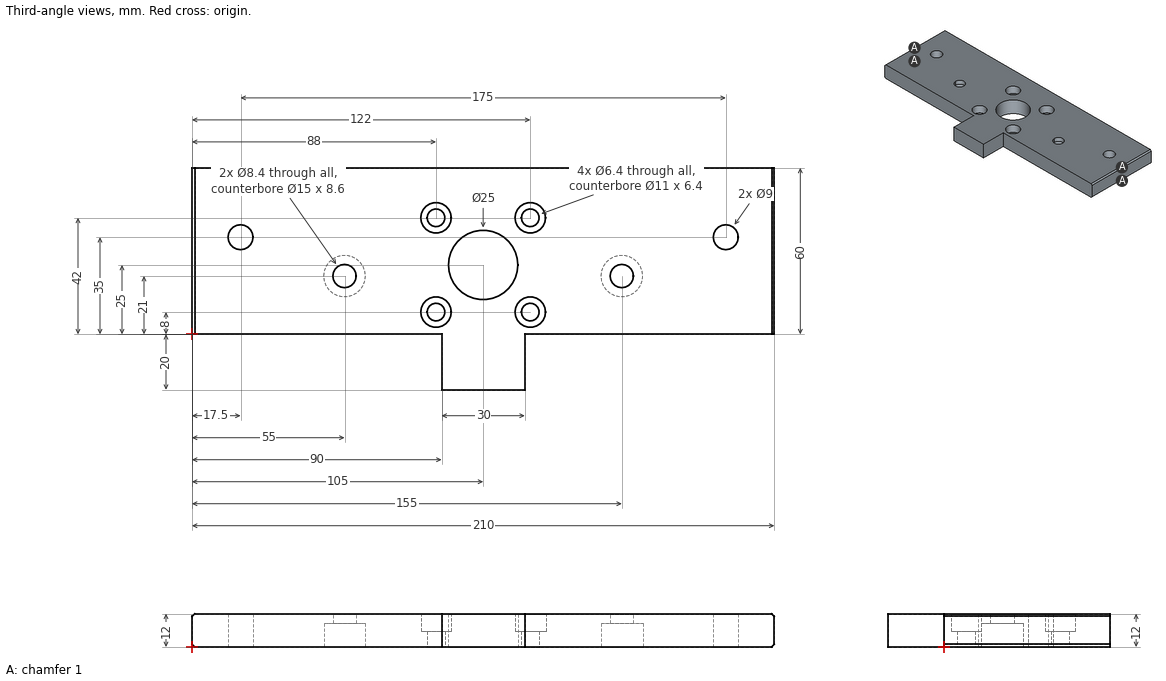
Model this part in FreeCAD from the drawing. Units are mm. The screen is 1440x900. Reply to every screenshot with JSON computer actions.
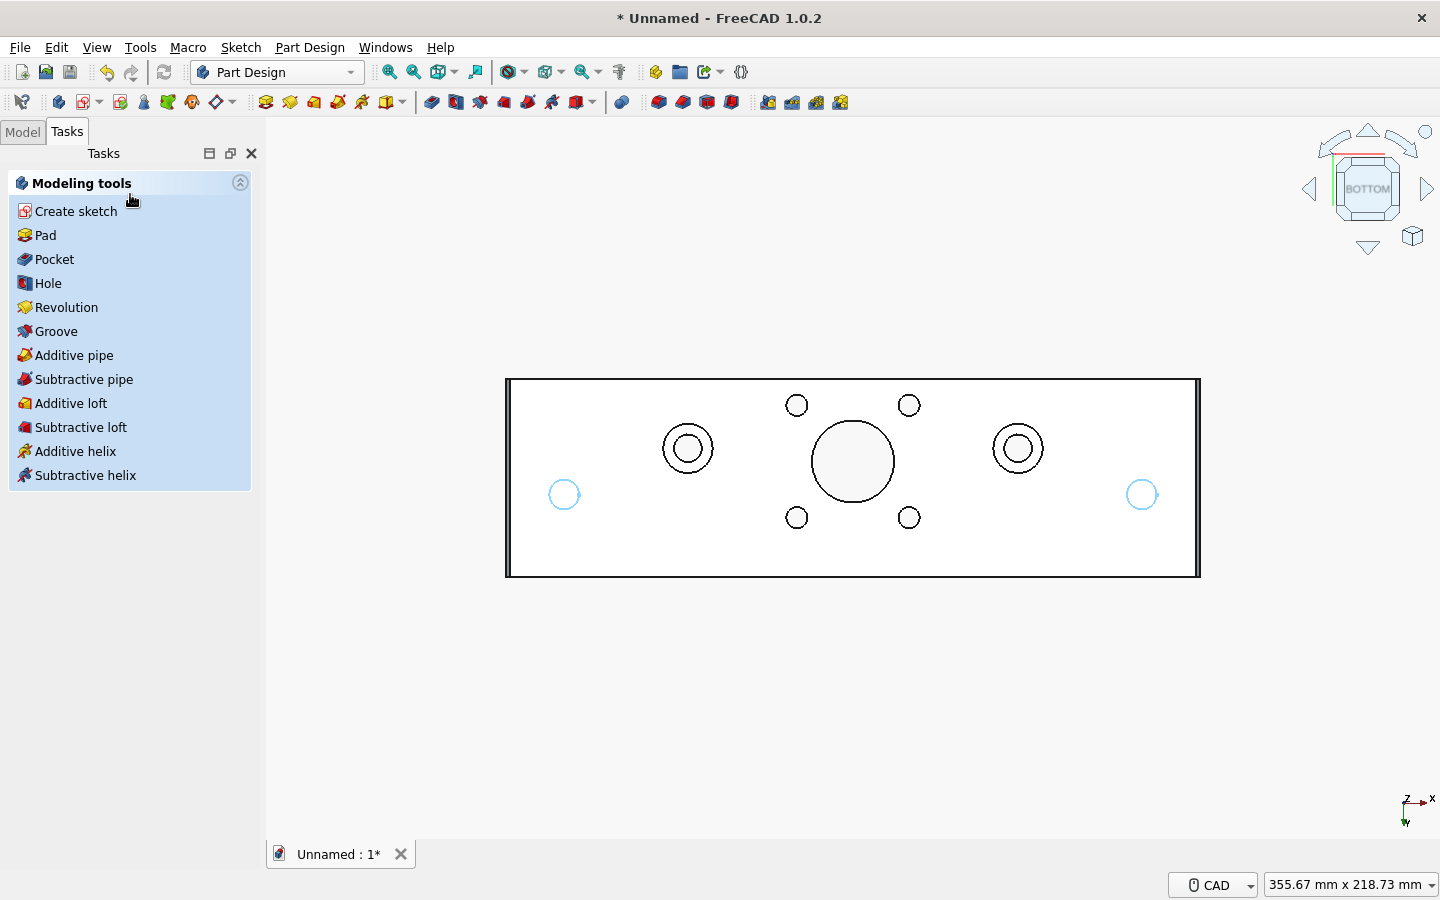
{"action": "left_click", "coordinate": [432, 102]}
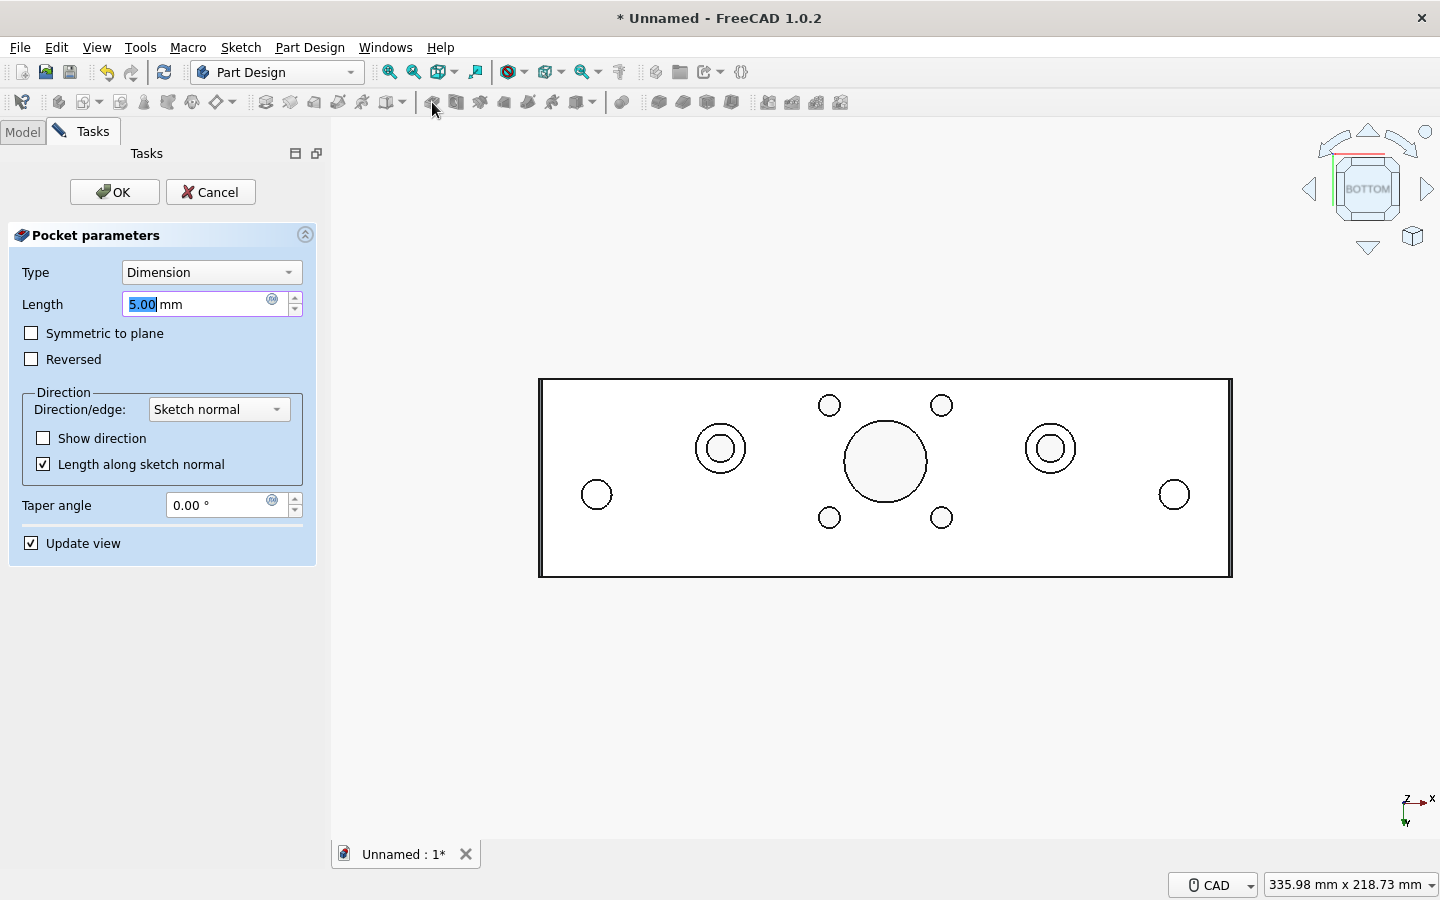
{"action": "left_click", "coordinate": [212, 272]}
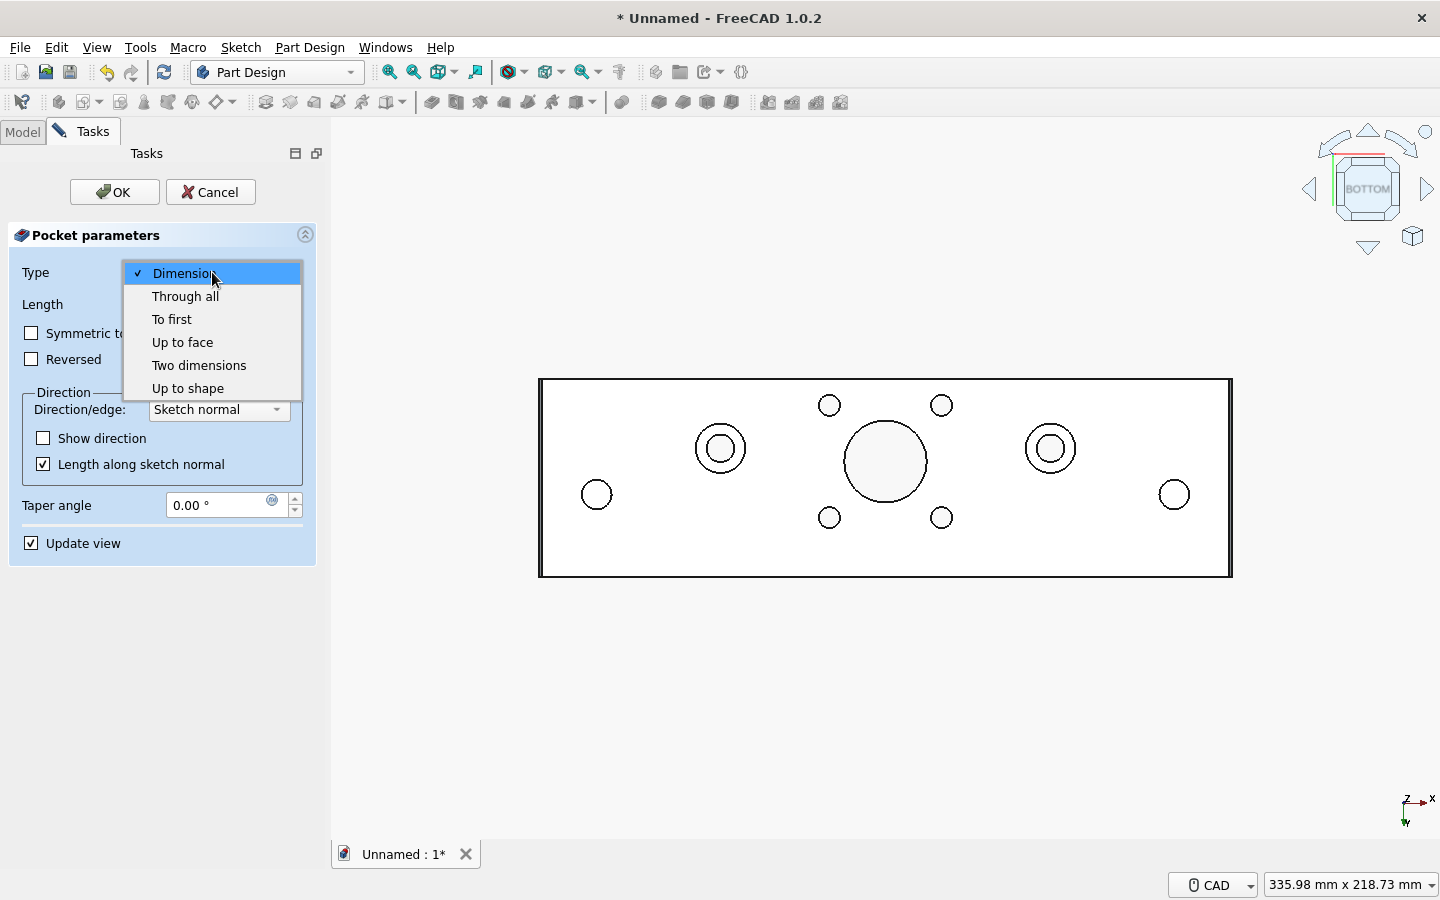
{"action": "left_click", "coordinate": [212, 296]}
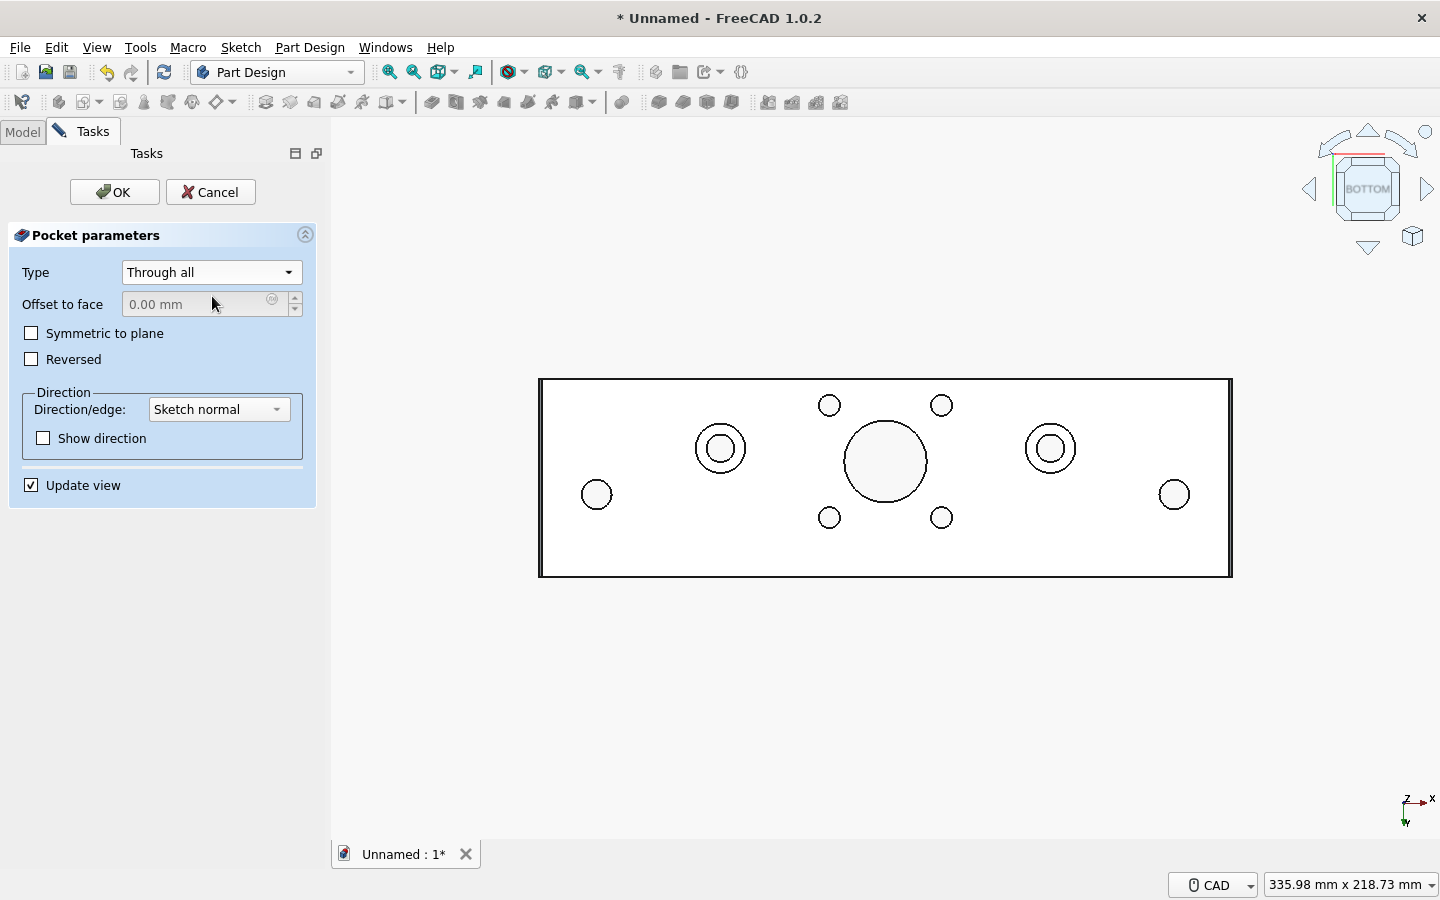
{"action": "left_click", "coordinate": [115, 192]}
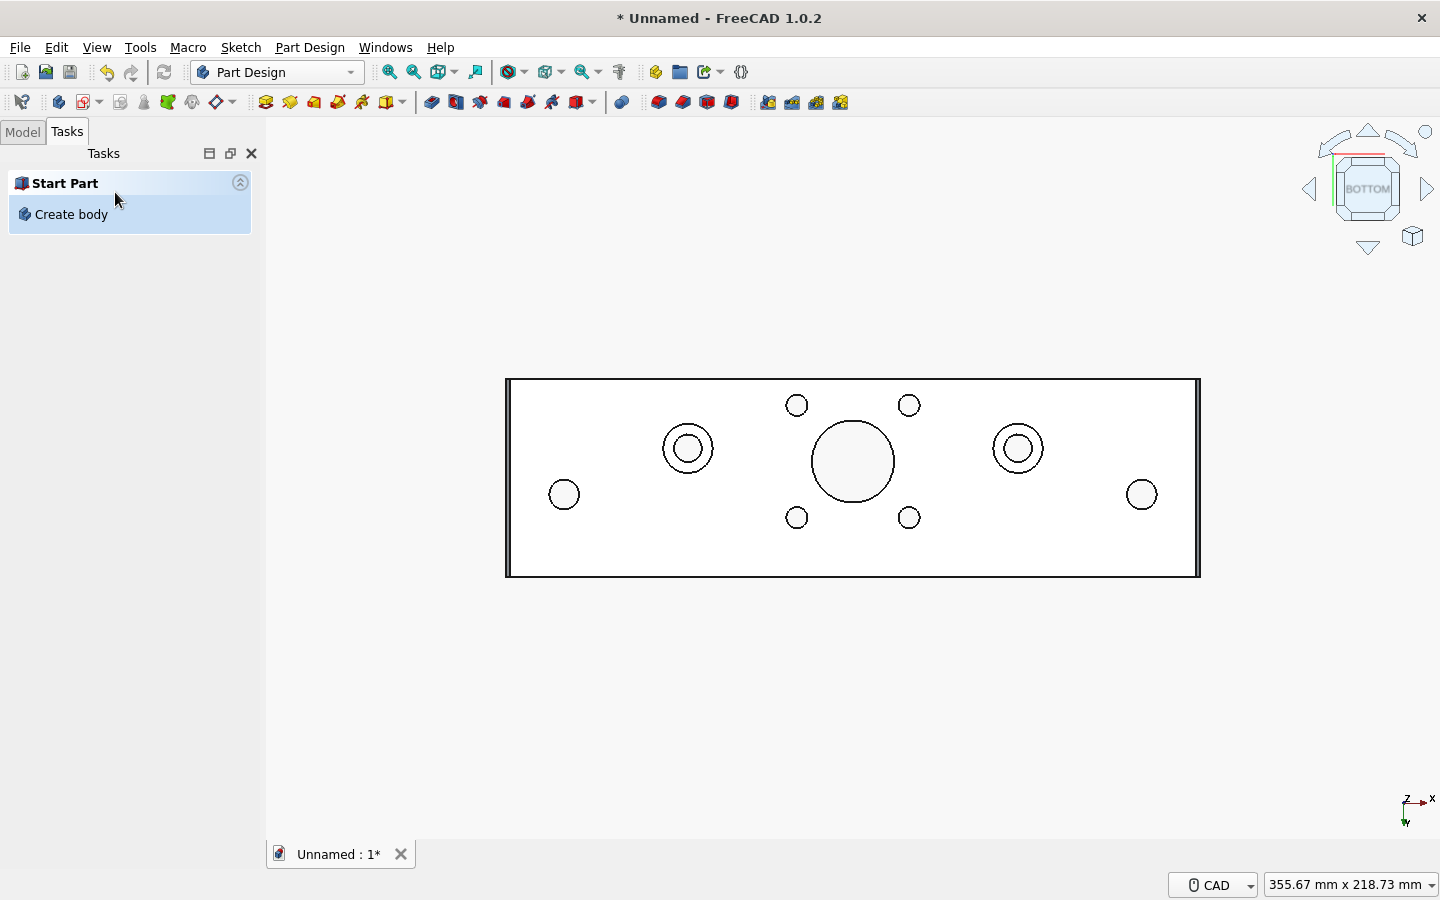
{"action": "left_click", "coordinate": [951, 477]}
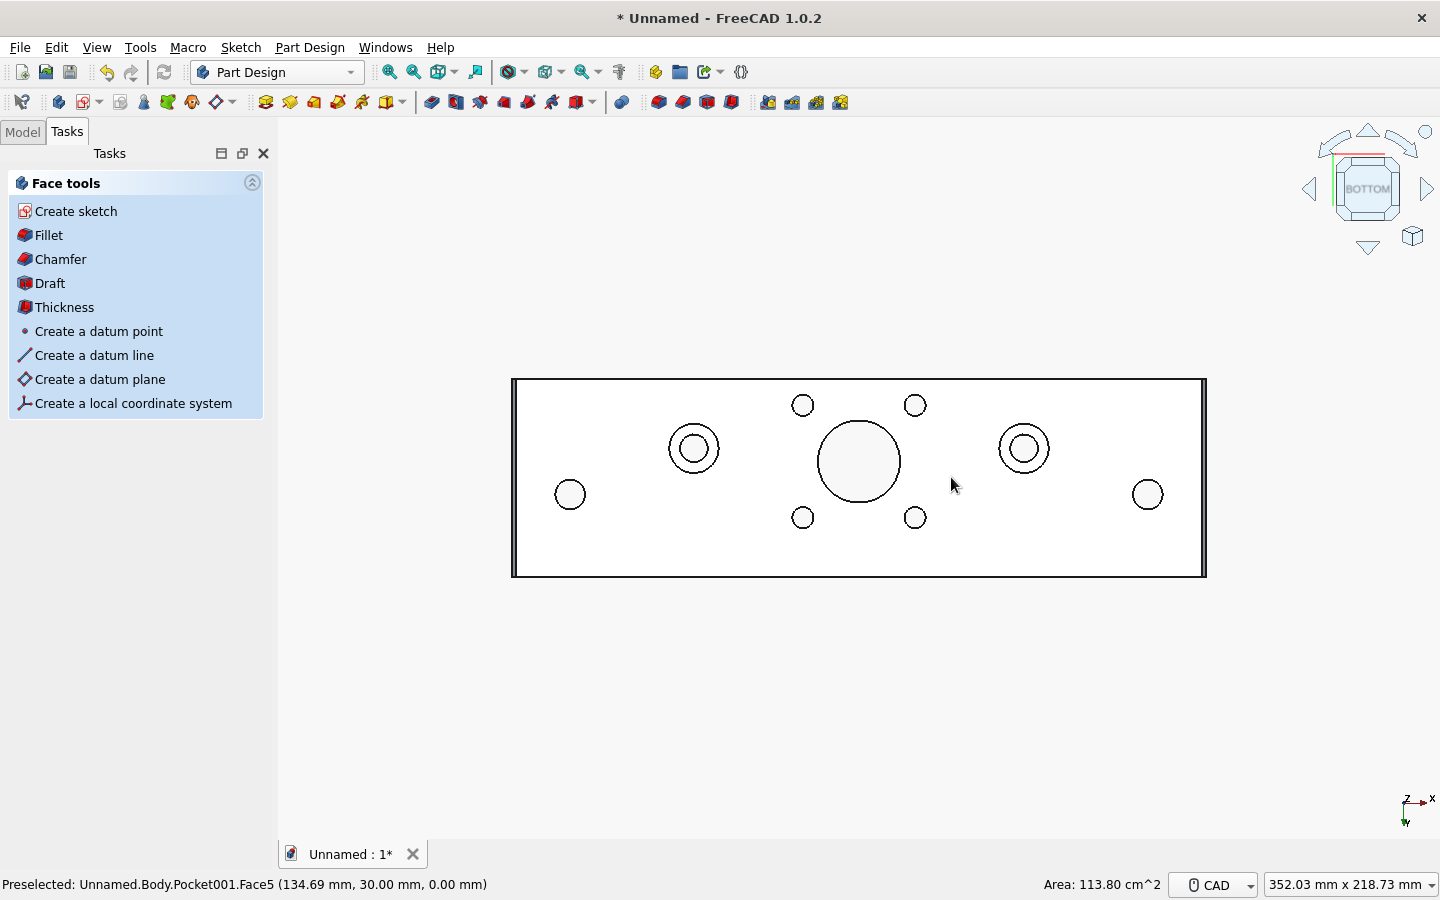
{"action": "left_click", "coordinate": [84, 102]}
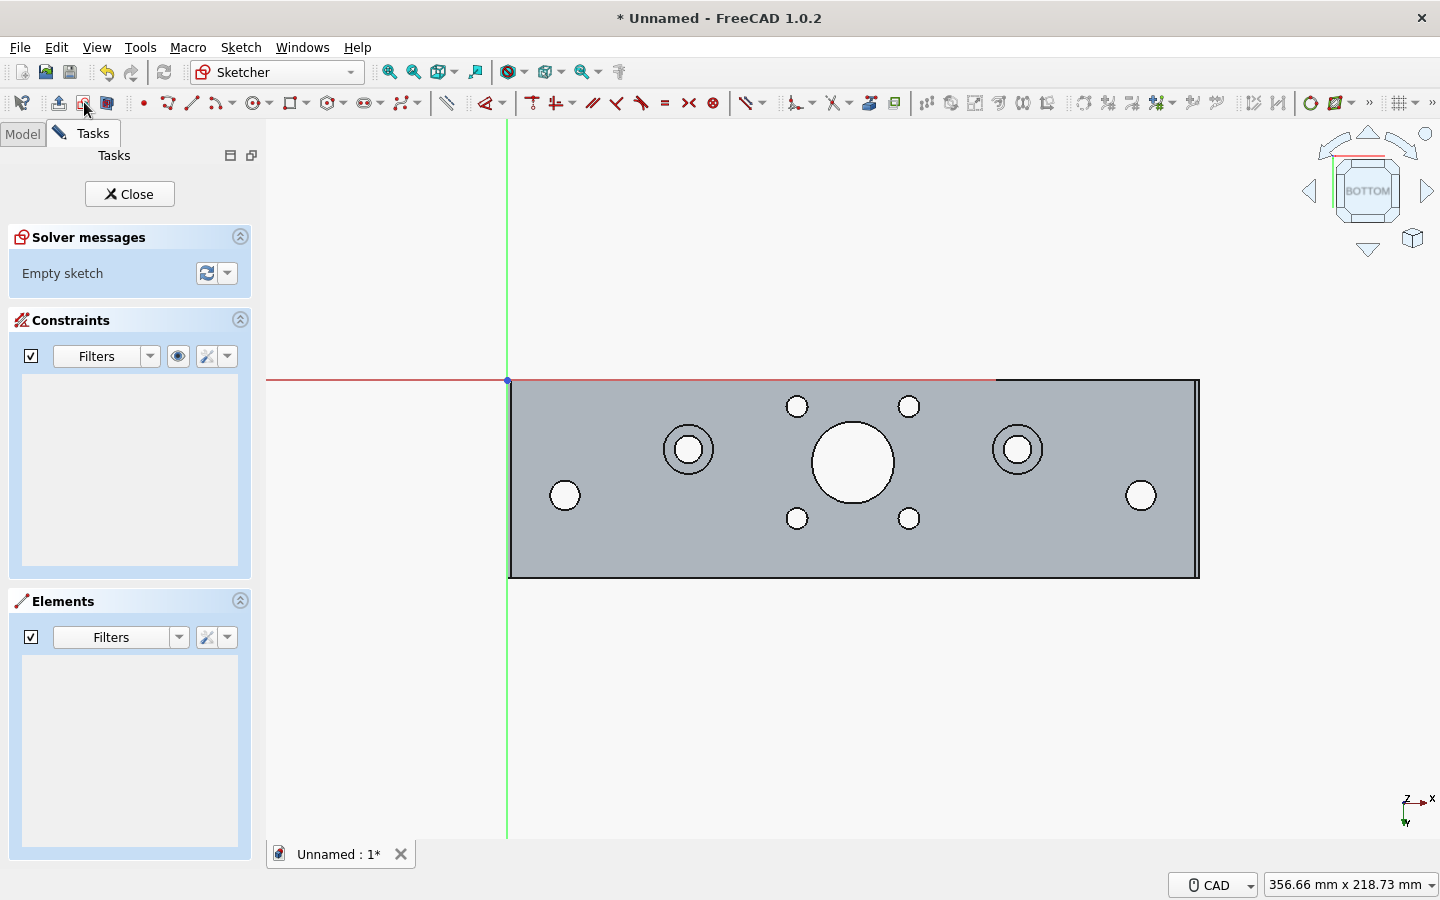
{"action": "scroll", "coordinate": [864, 327], "scroll_direction": "up", "scroll_amount": 10}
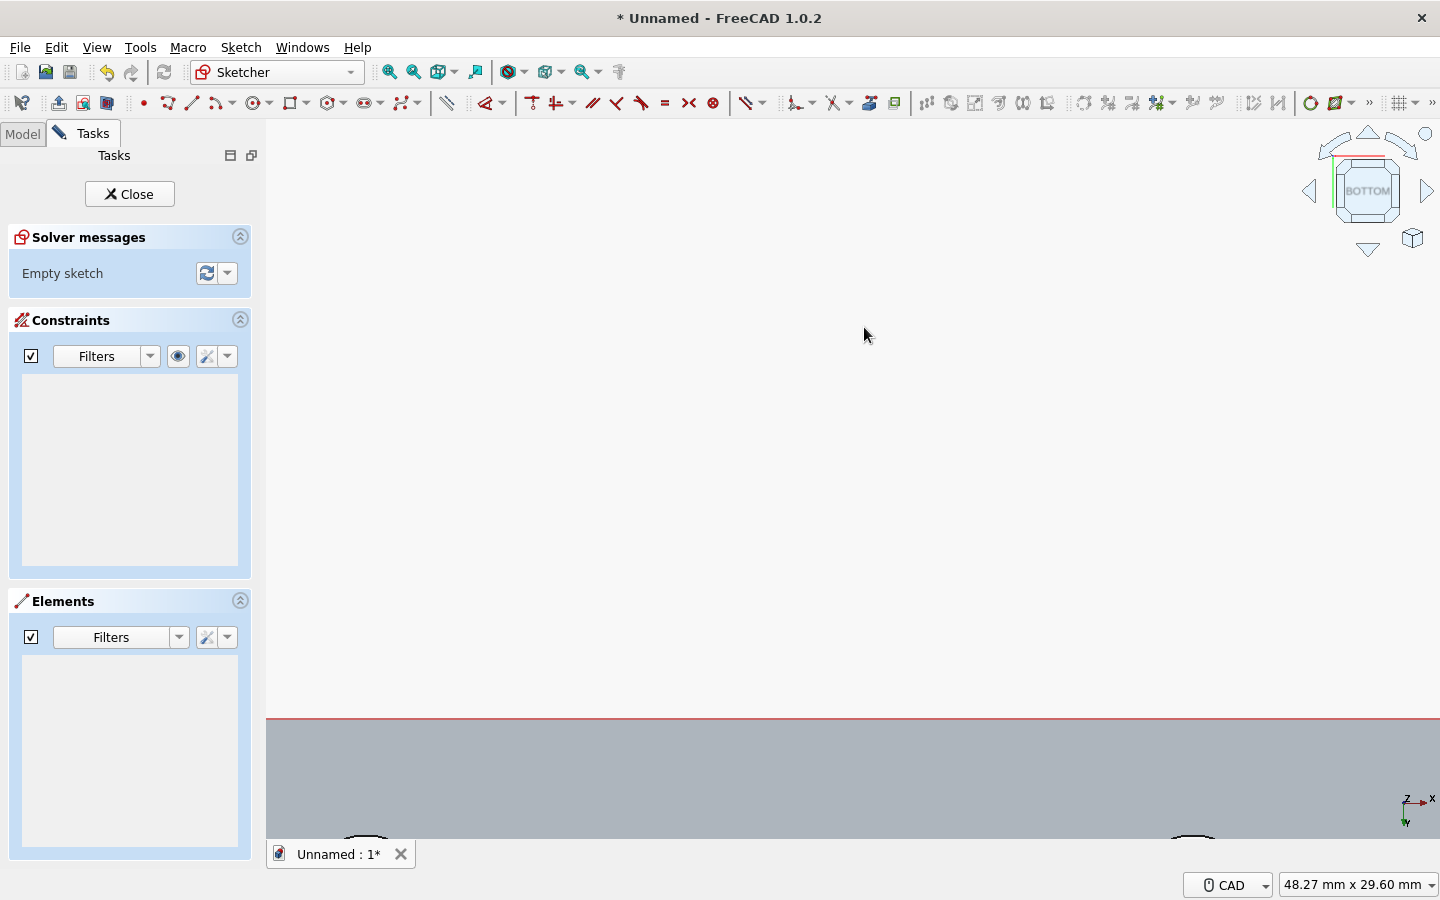
{"action": "key", "text": "g r"}